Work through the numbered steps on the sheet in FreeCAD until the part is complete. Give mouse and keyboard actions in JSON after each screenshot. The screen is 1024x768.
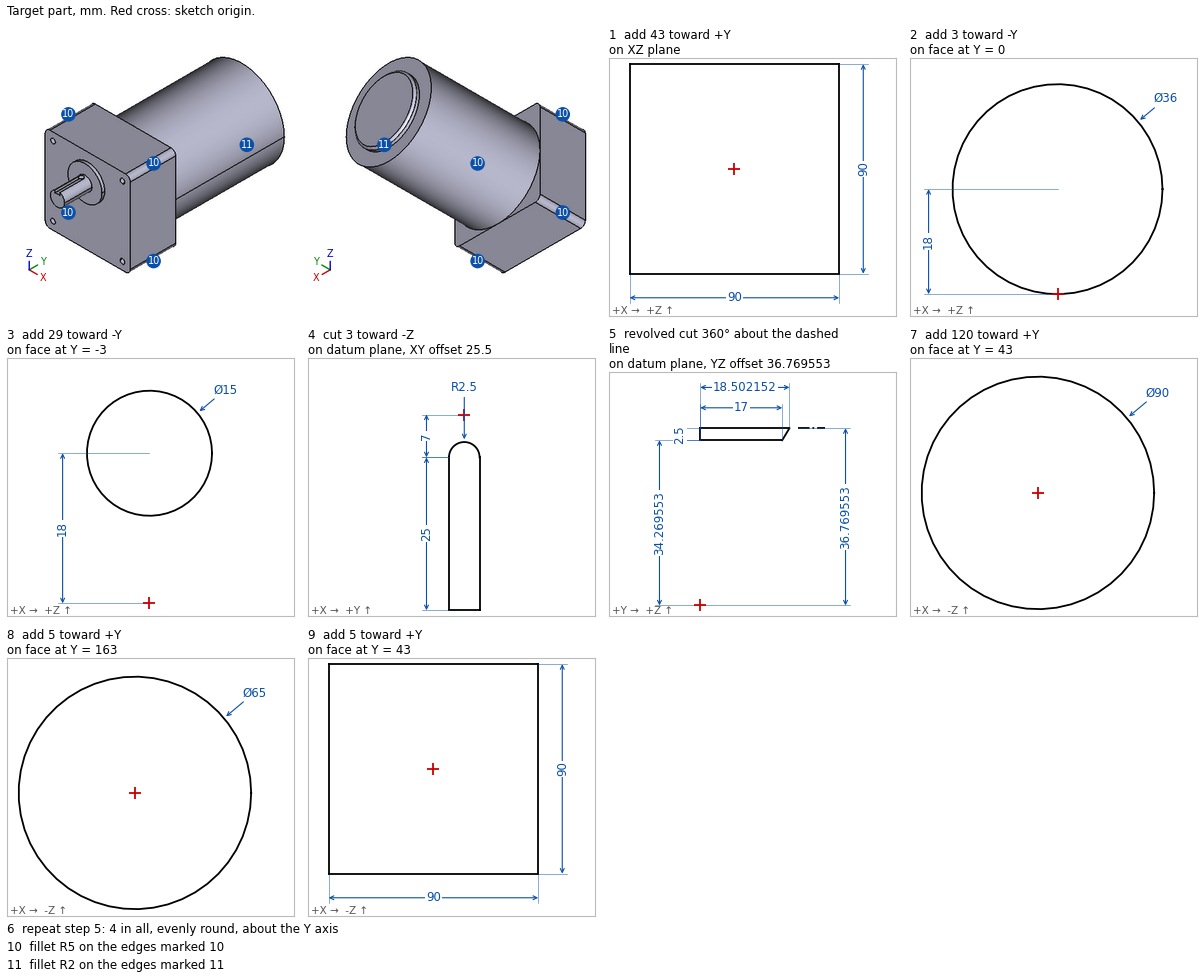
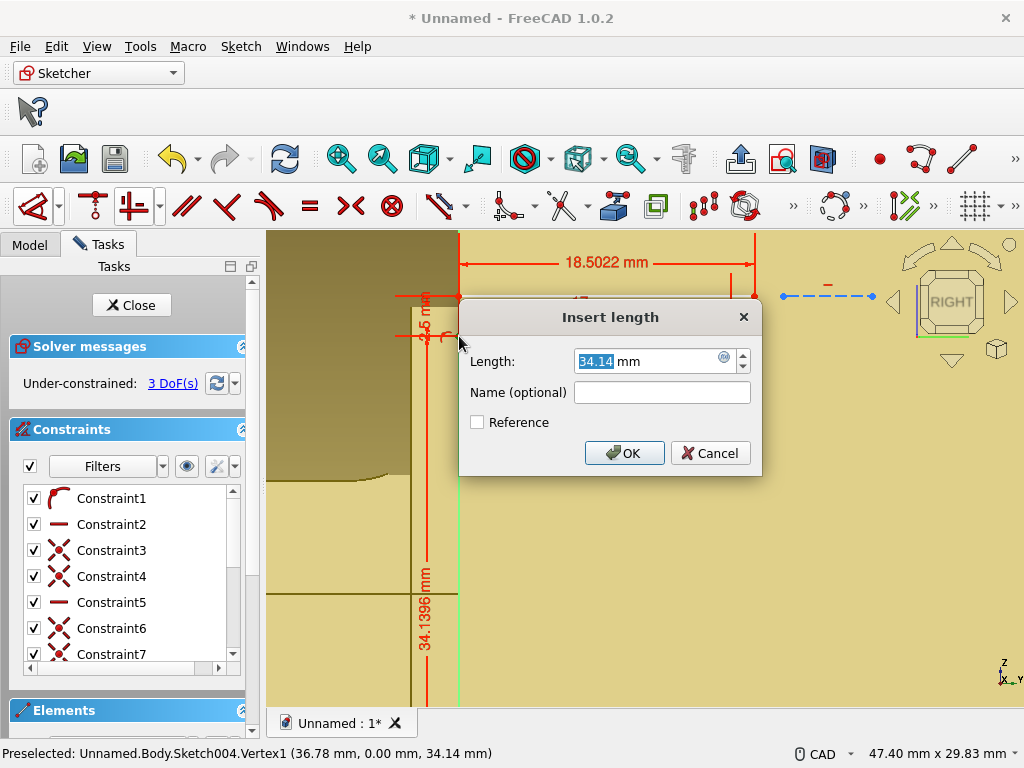
{"action": "type", "text": "34.269553"}
{"action": "key", "text": "Return"}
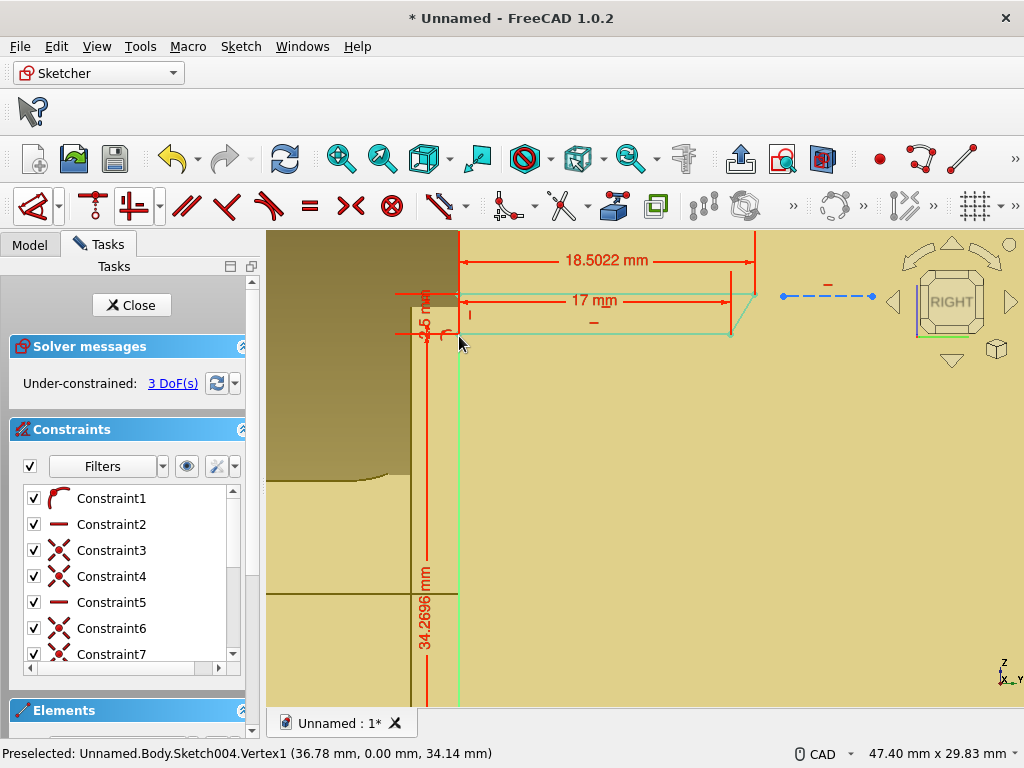
{"action": "left_click", "coordinate": [784, 296]}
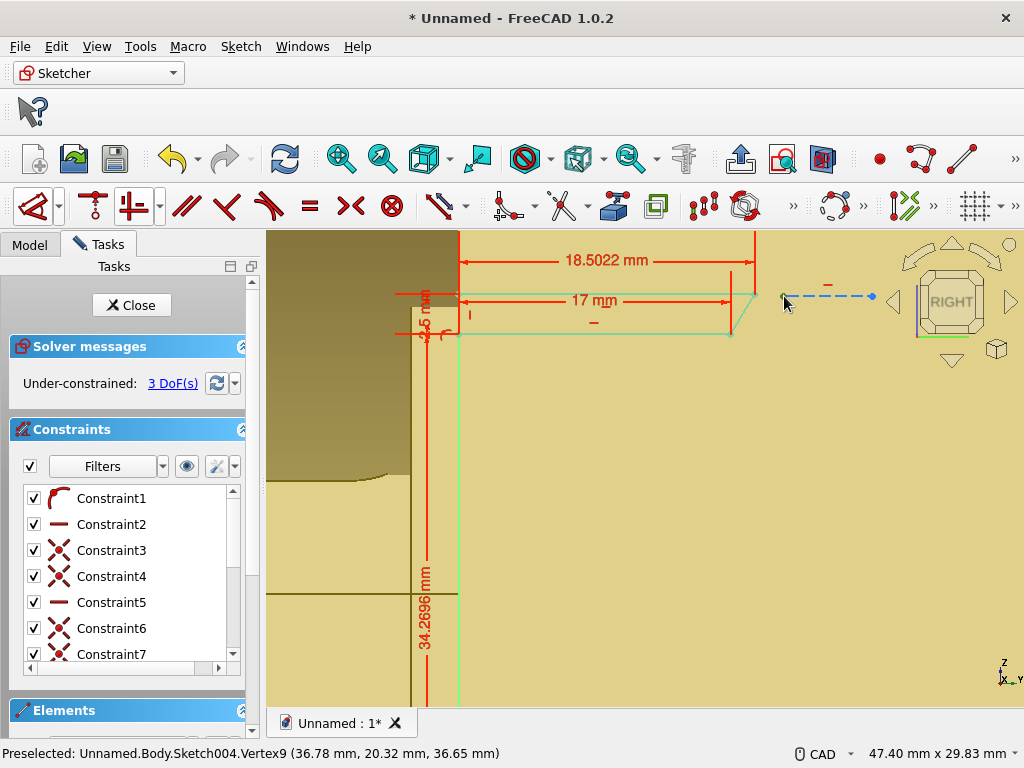
{"action": "left_click", "coordinate": [58, 206]}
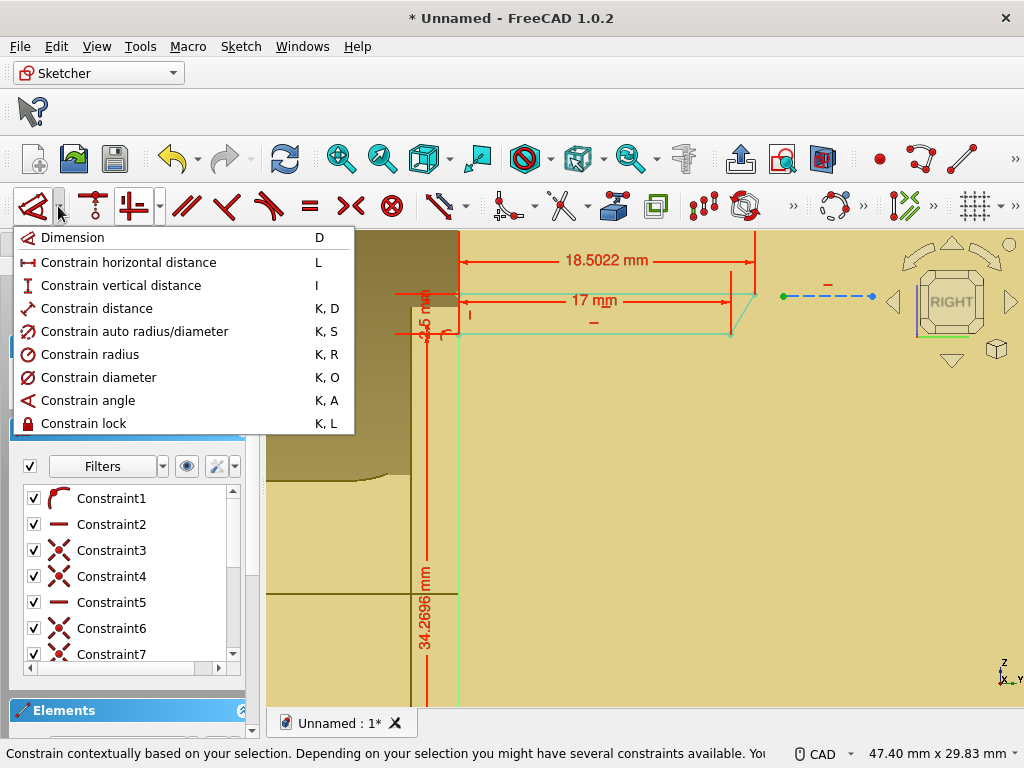
{"action": "left_click", "coordinate": [184, 286]}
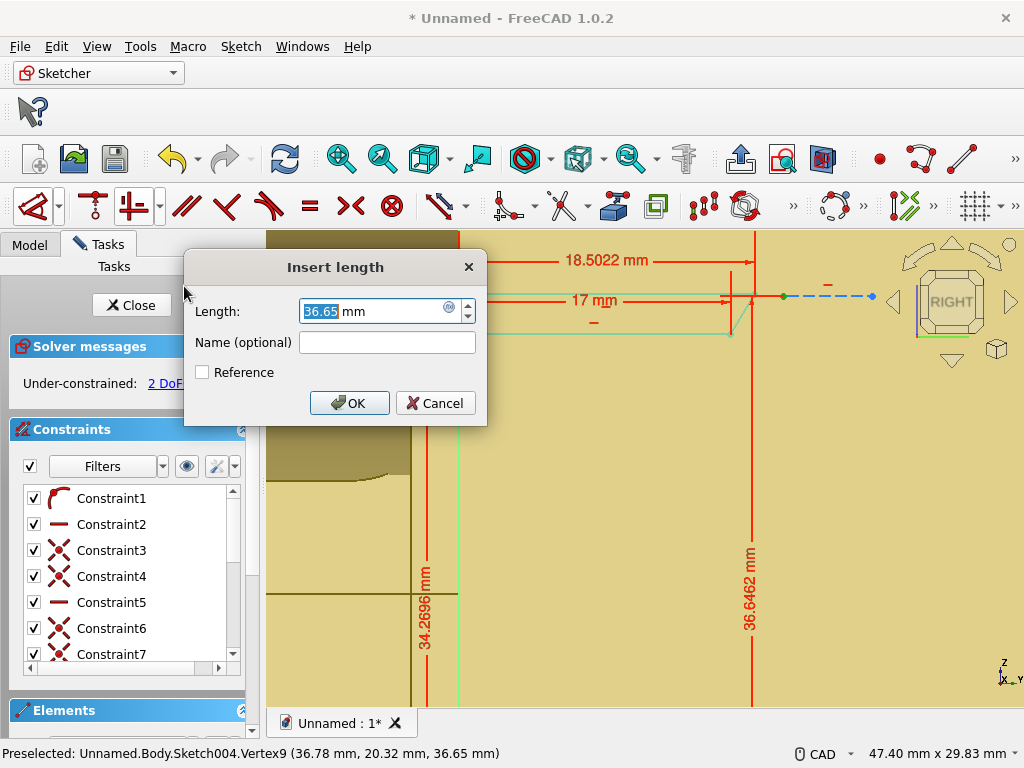
{"action": "type", "text": "36.769553"}
{"action": "key", "text": "Return"}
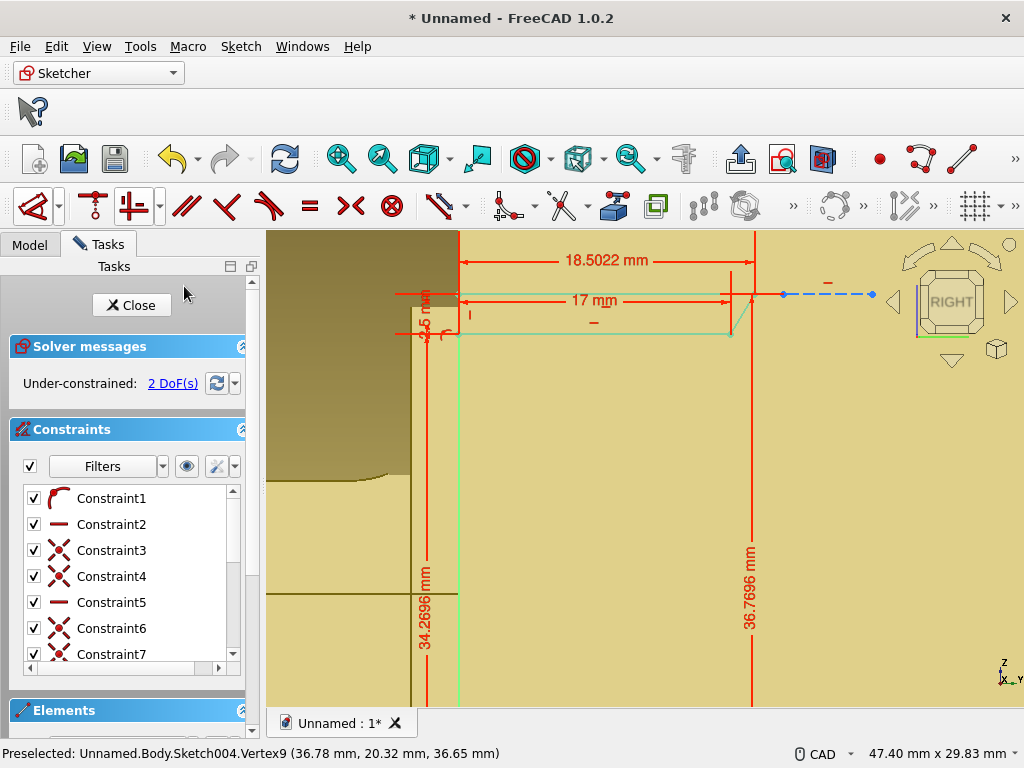
{"action": "left_click", "coordinate": [132, 305]}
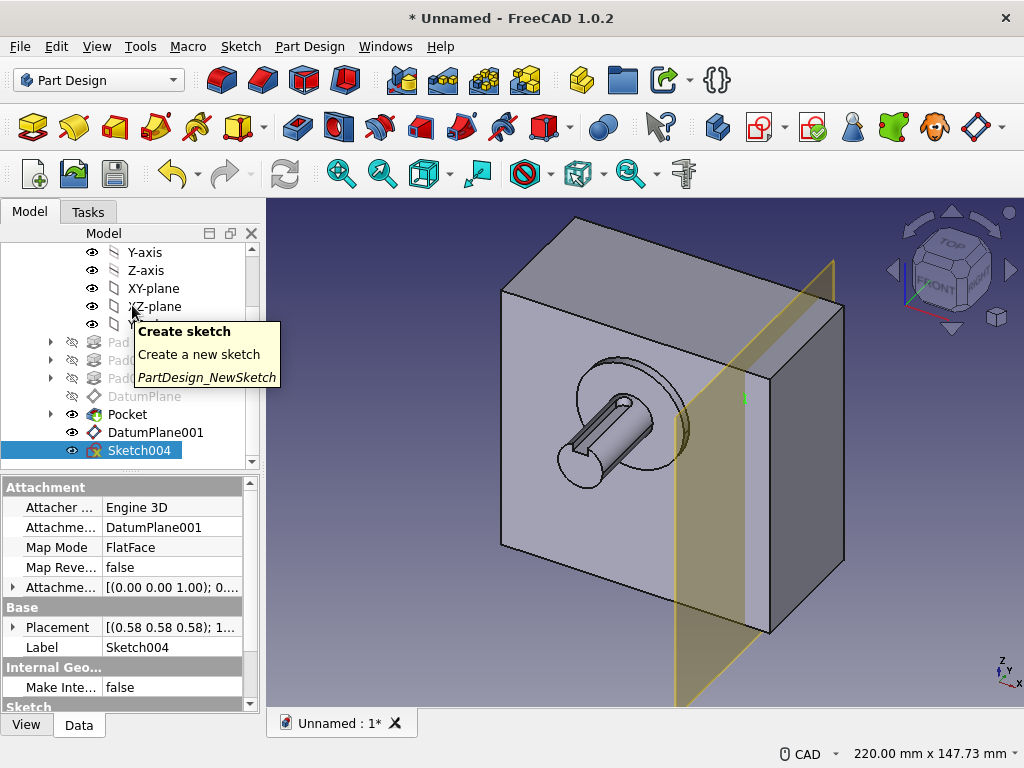
{"action": "left_click", "coordinate": [380, 128]}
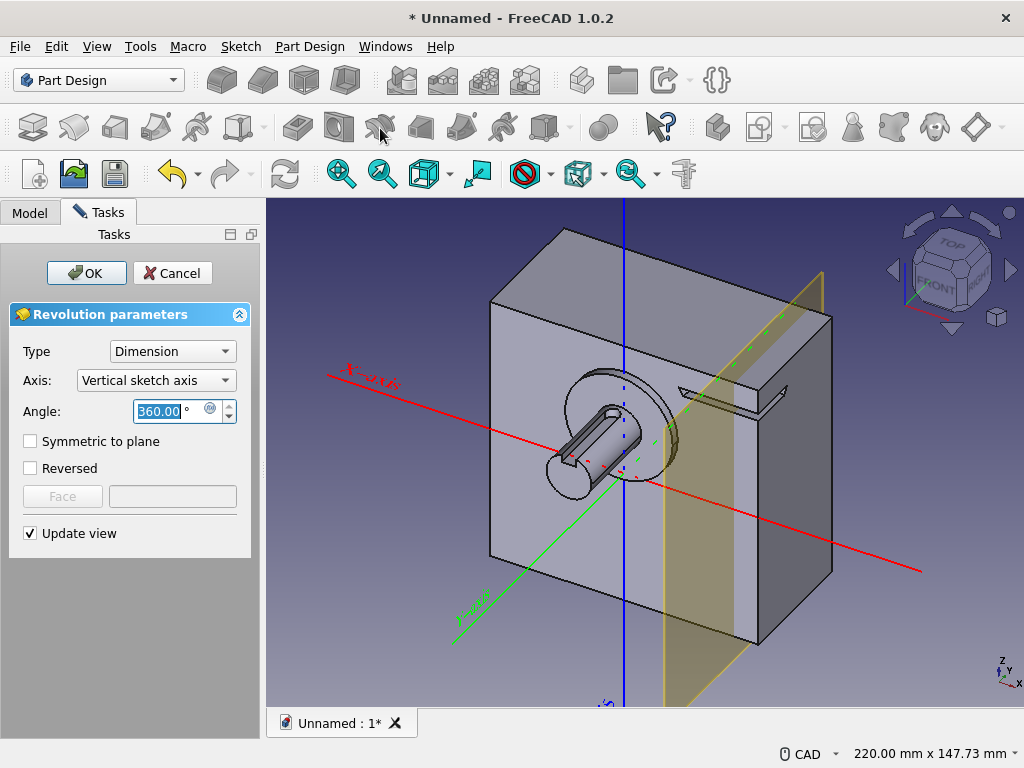
{"action": "left_click", "coordinate": [157, 380]}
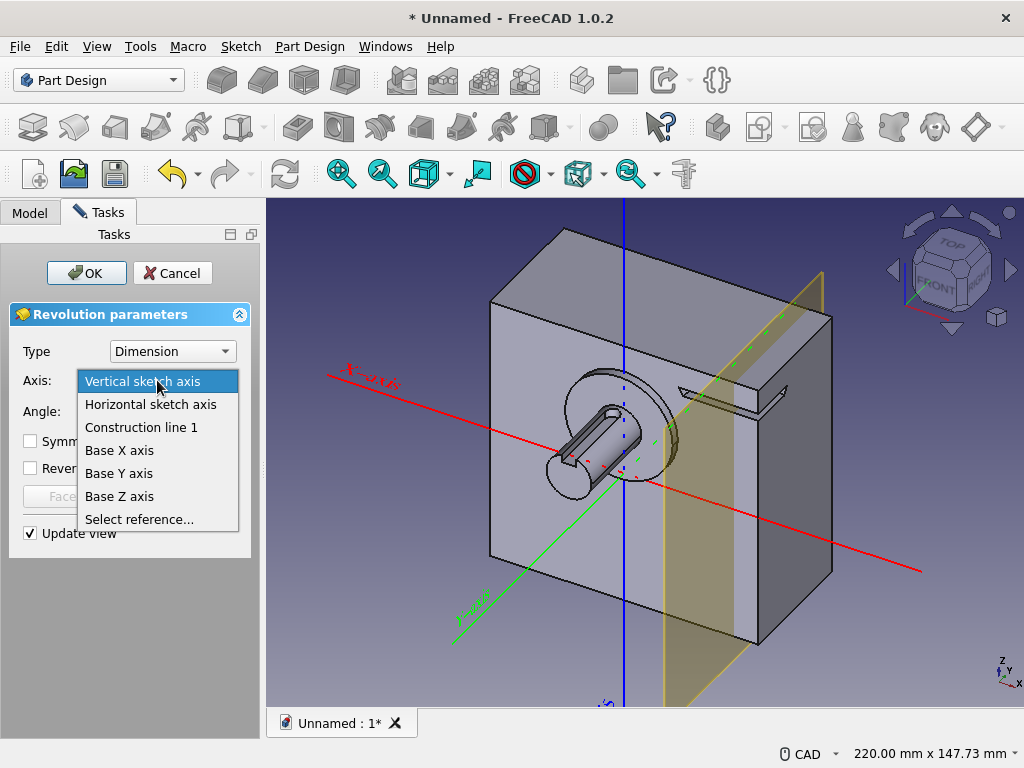
{"action": "left_click", "coordinate": [156, 428]}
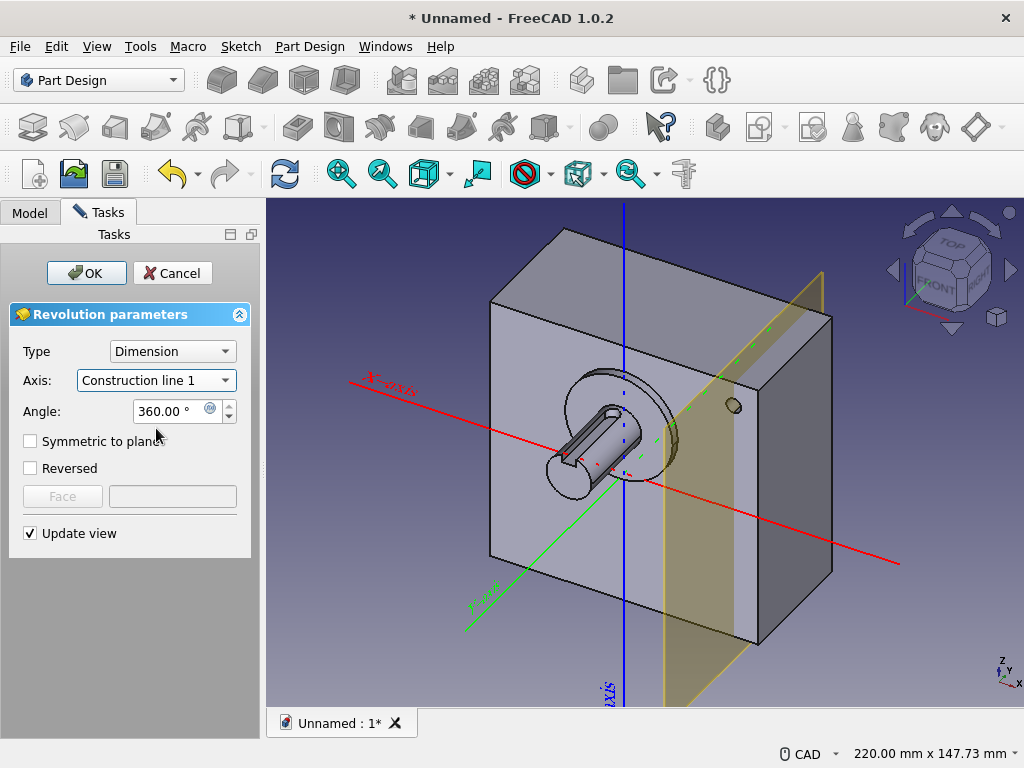
{"action": "left_click", "coordinate": [87, 273]}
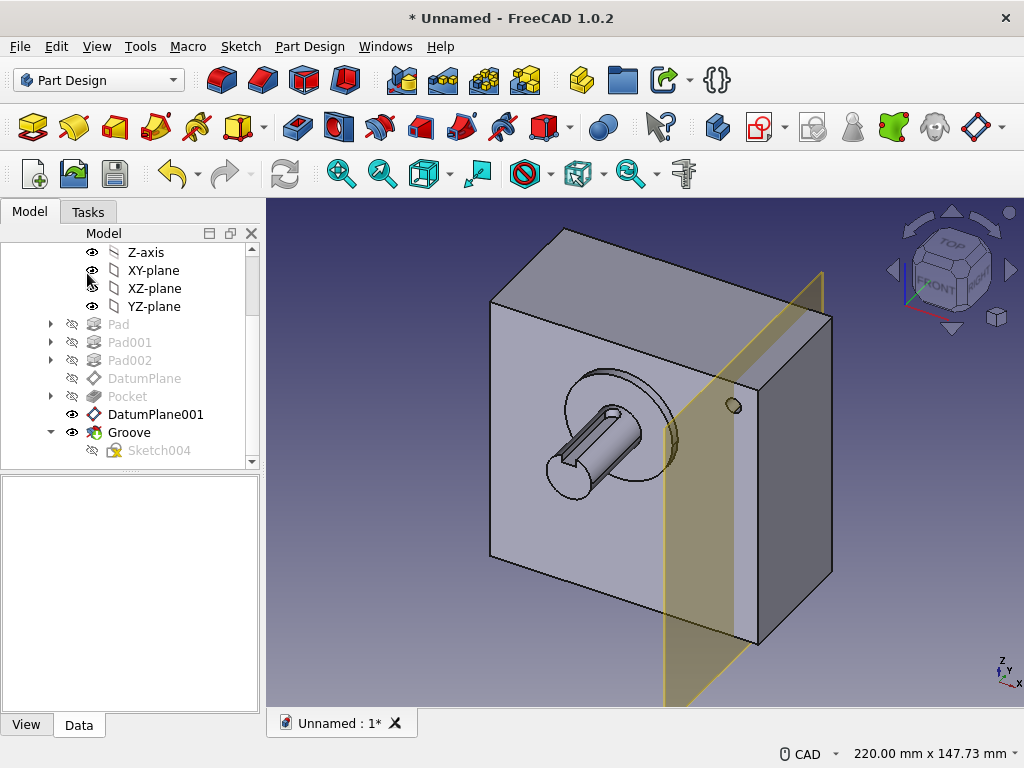
{"action": "left_click", "coordinate": [117, 414]}
{"action": "key", "text": "space"}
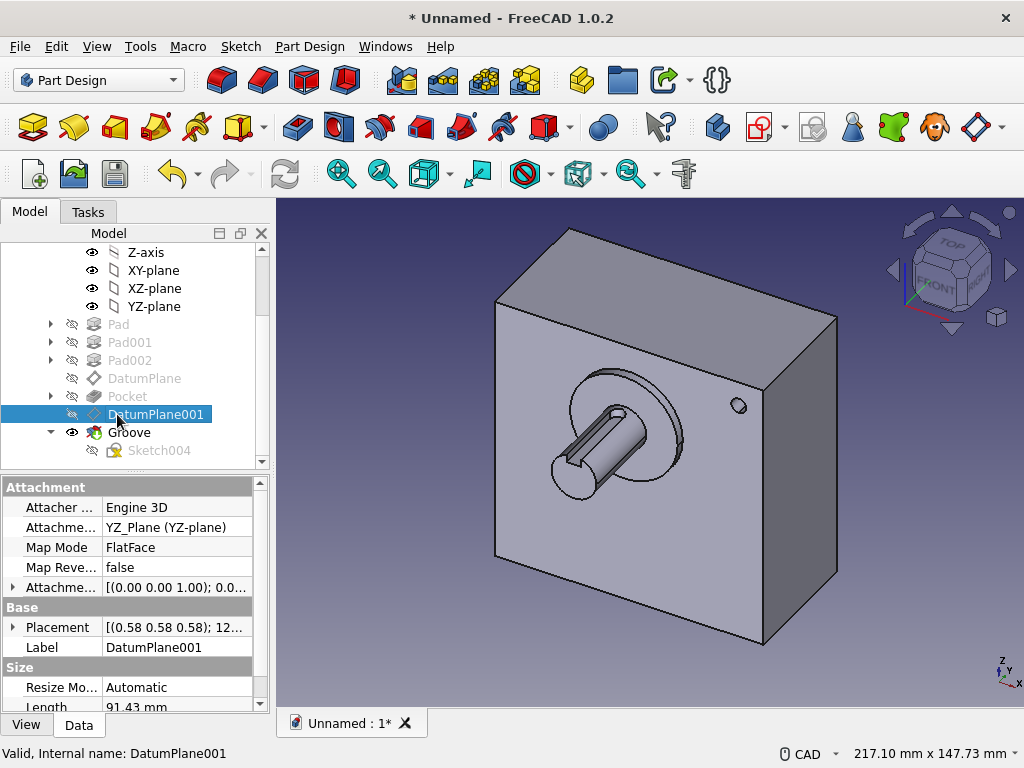
{"action": "left_click", "coordinate": [117, 432]}